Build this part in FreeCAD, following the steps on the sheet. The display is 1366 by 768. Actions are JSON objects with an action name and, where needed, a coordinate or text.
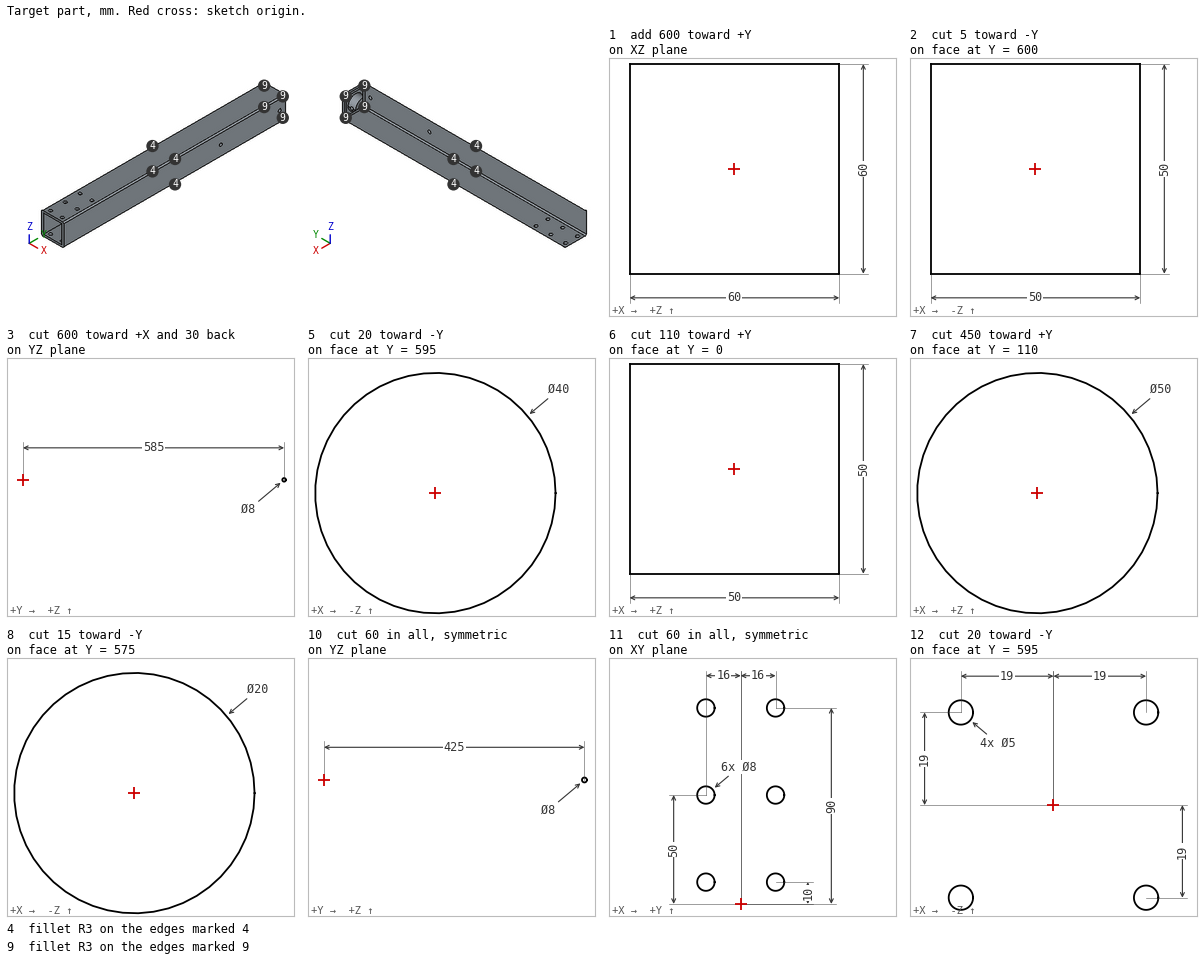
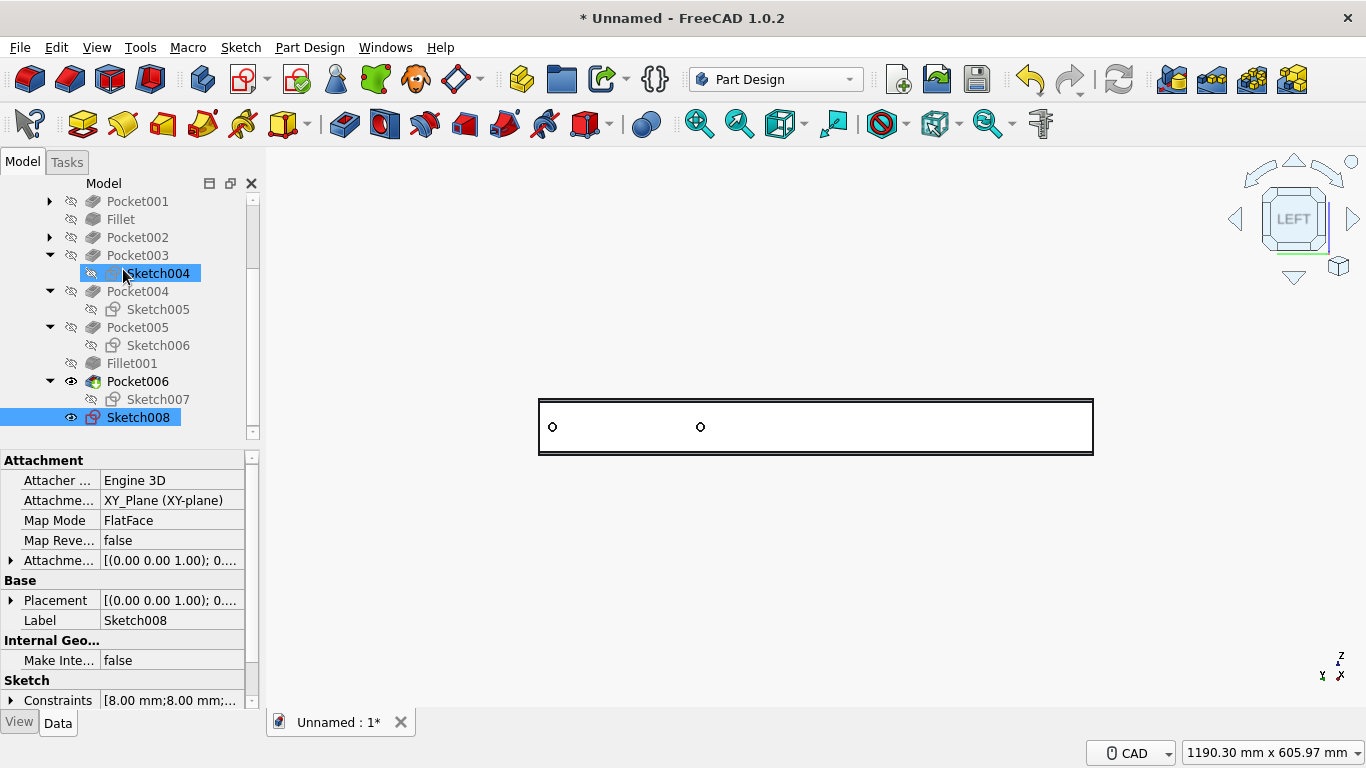
{"action": "left_click", "coordinate": [346, 124]}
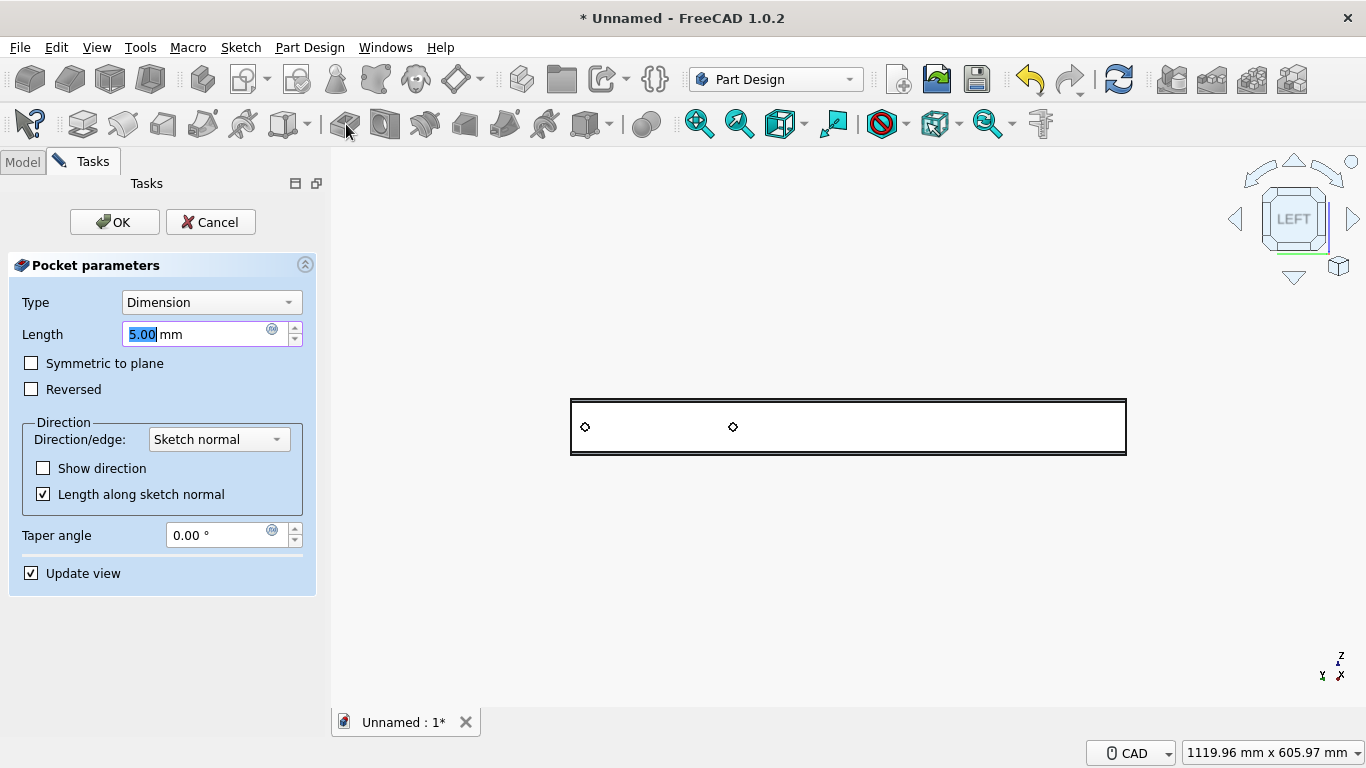
{"action": "type", "text": "60"}
{"action": "key", "text": "Tab"}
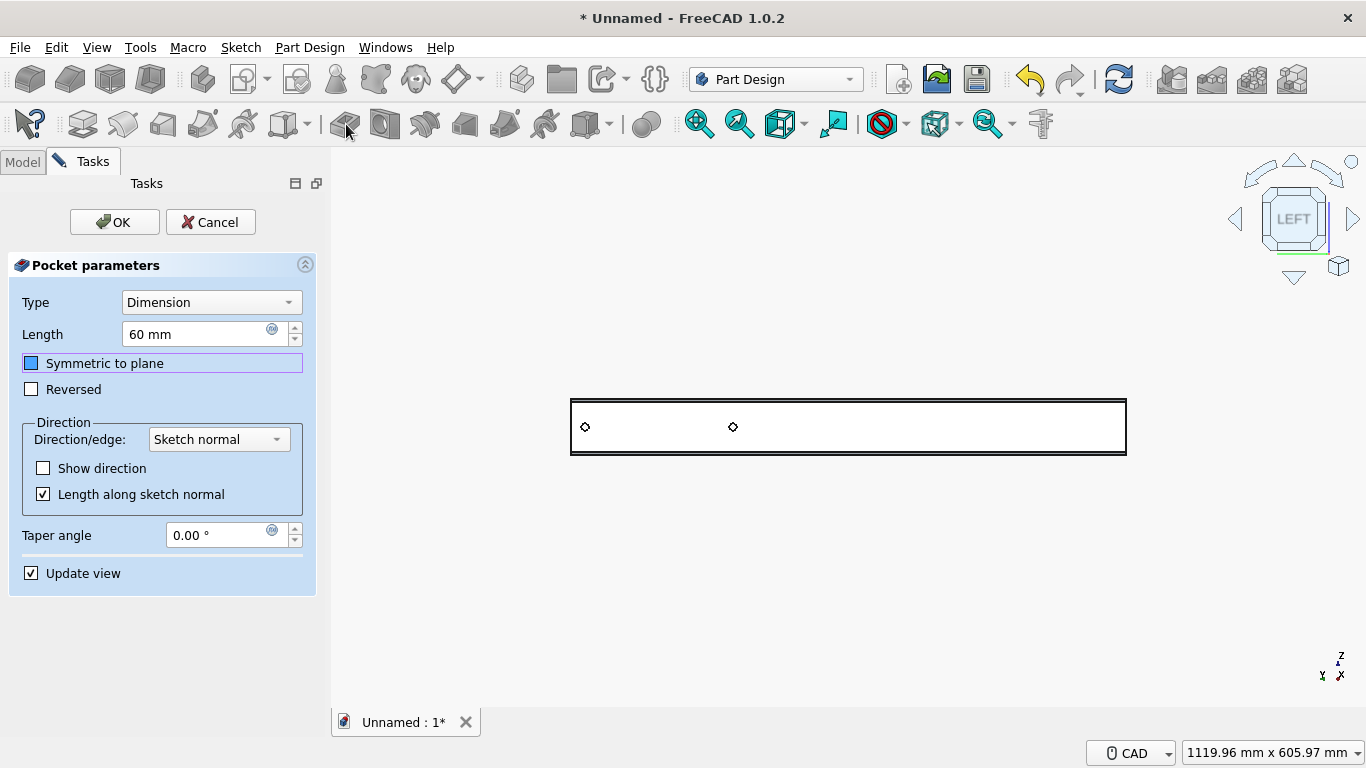
{"action": "left_click", "coordinate": [30, 363]}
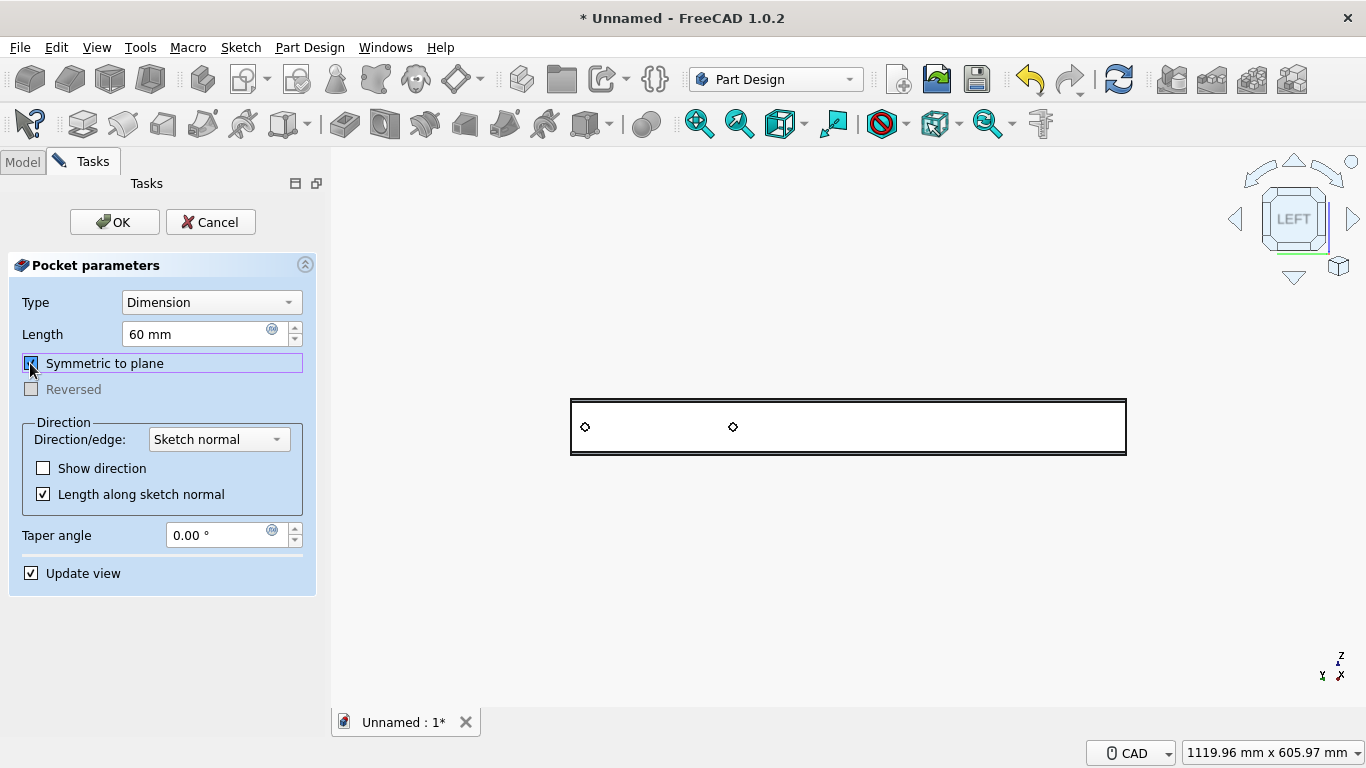
{"action": "left_click", "coordinate": [115, 222]}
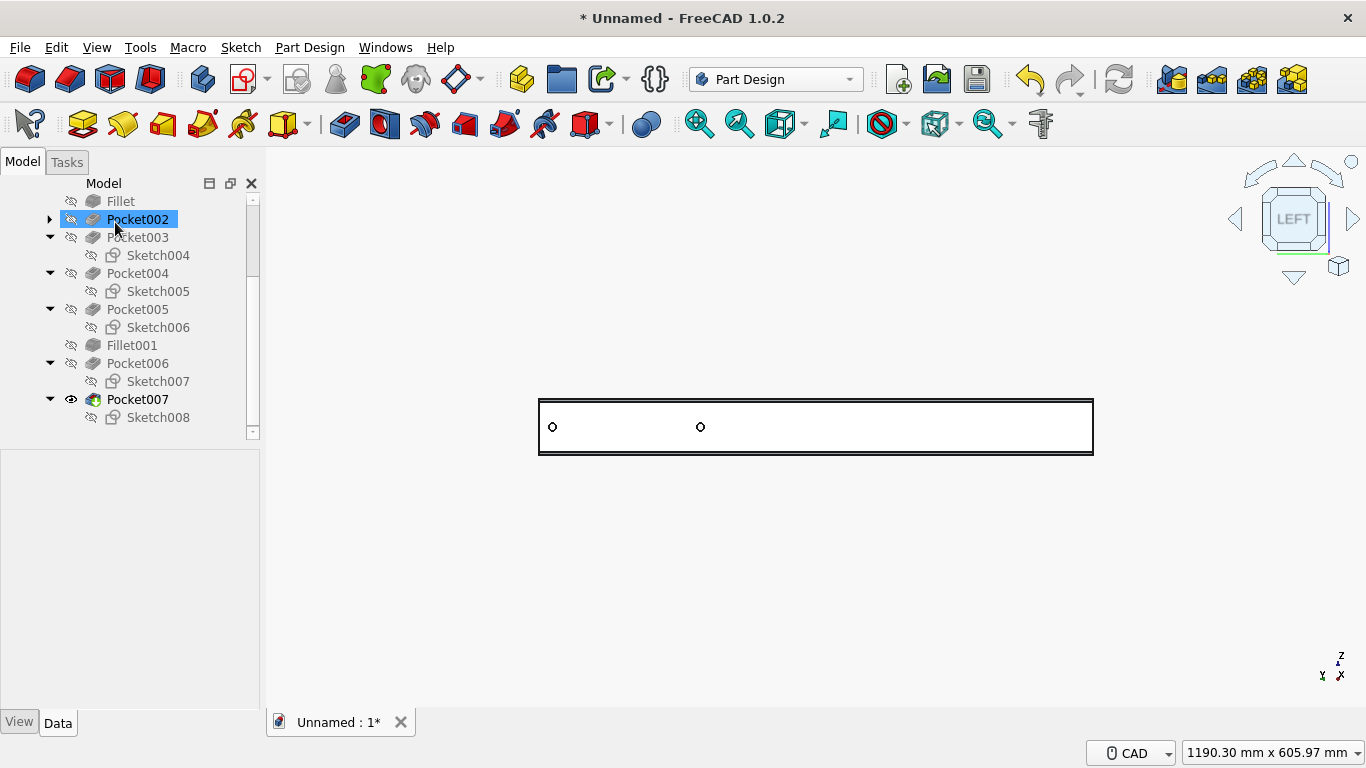
{"action": "key", "text": "4"}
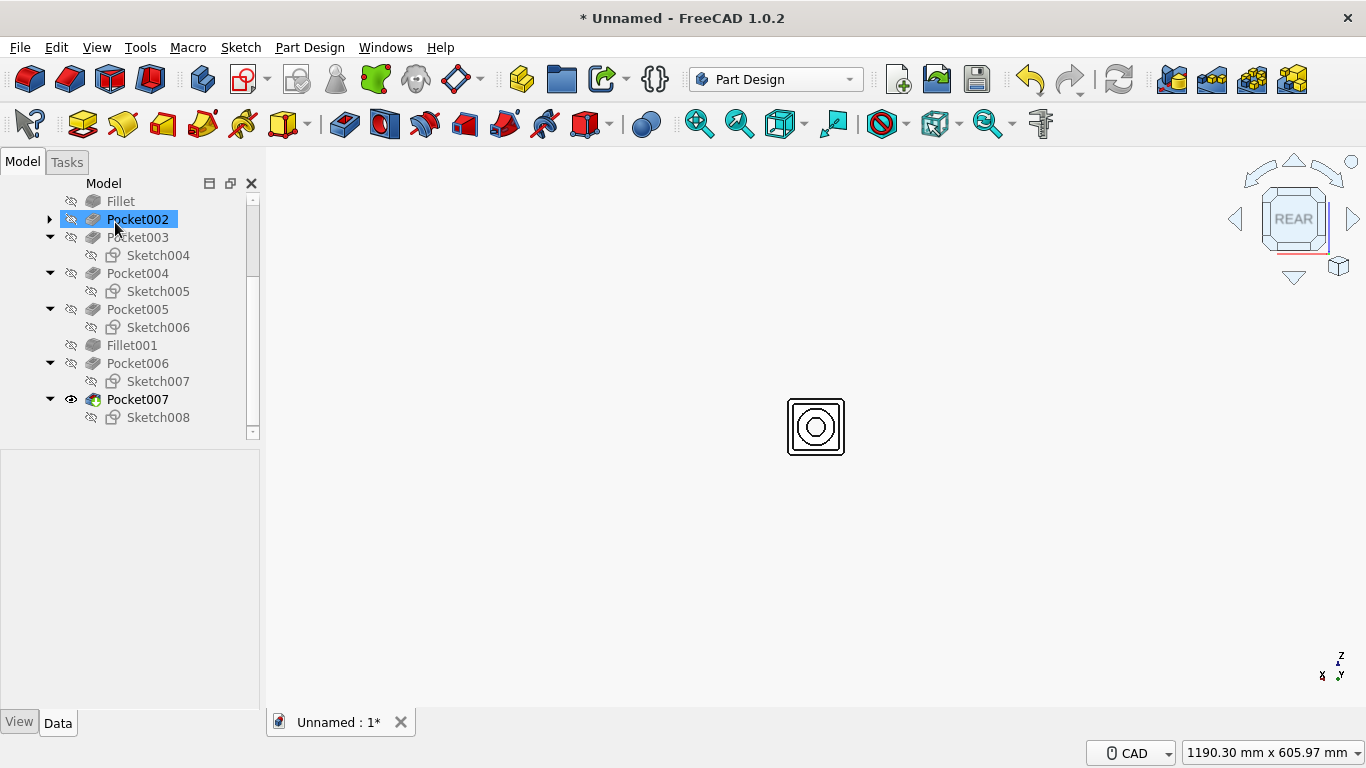
{"action": "left_click", "coordinate": [700, 124]}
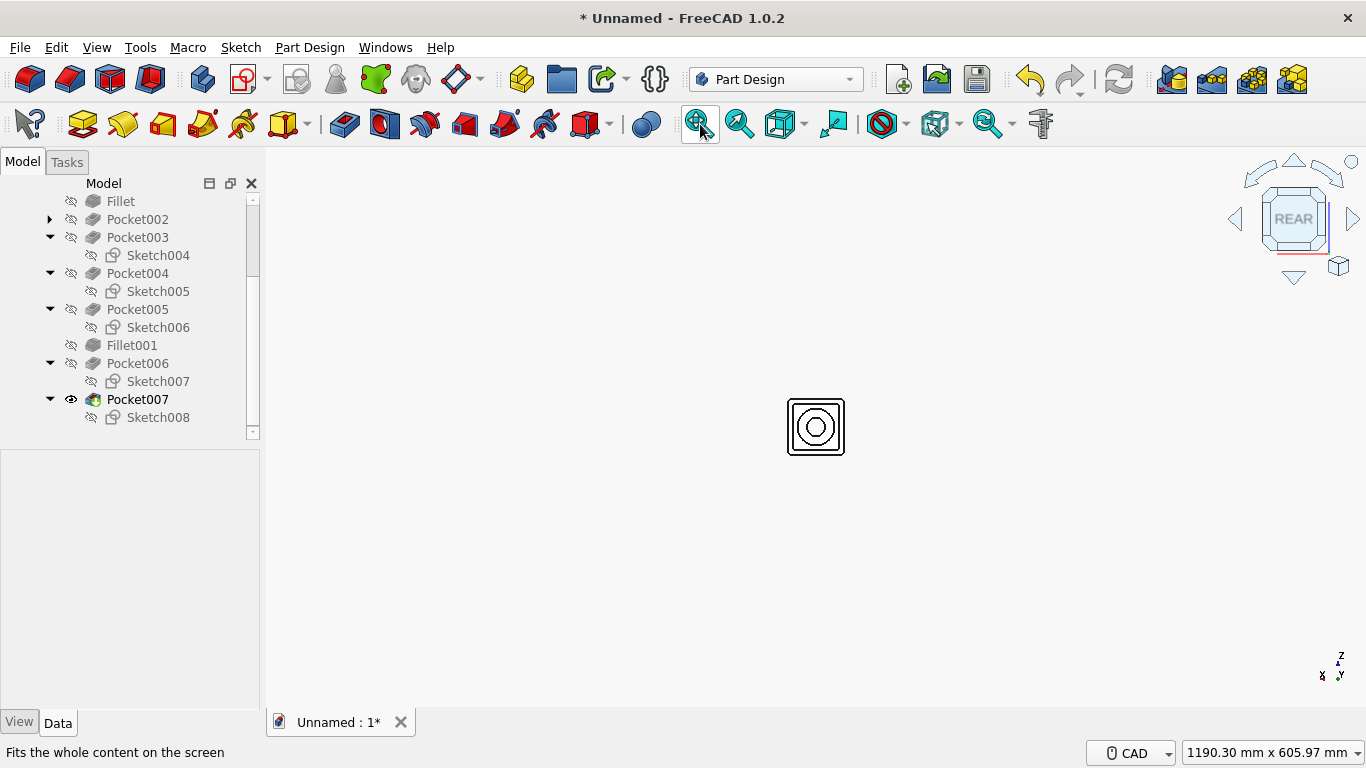
{"action": "scroll", "coordinate": [796, 406], "scroll_direction": "up", "scroll_amount": 7}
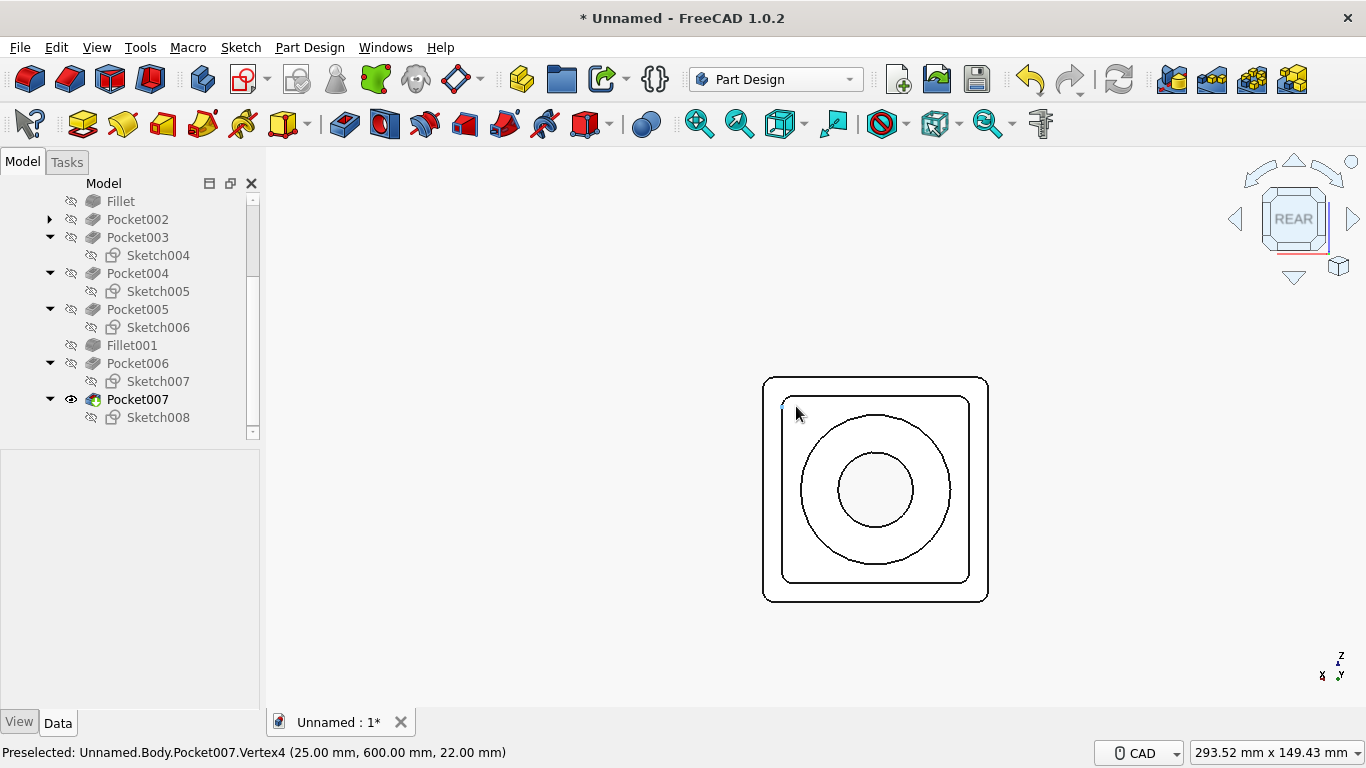
{"action": "left_click", "coordinate": [795, 408]}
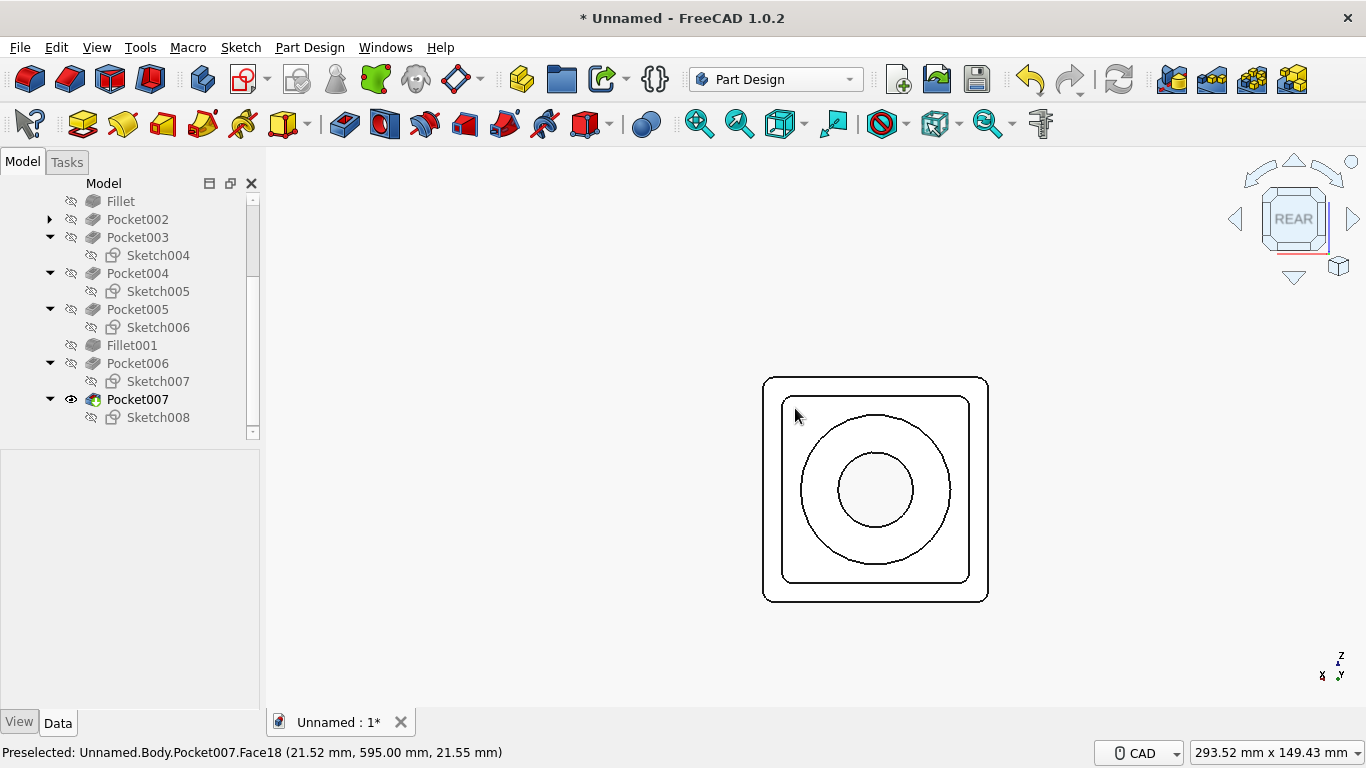
{"action": "left_click", "coordinate": [244, 80]}